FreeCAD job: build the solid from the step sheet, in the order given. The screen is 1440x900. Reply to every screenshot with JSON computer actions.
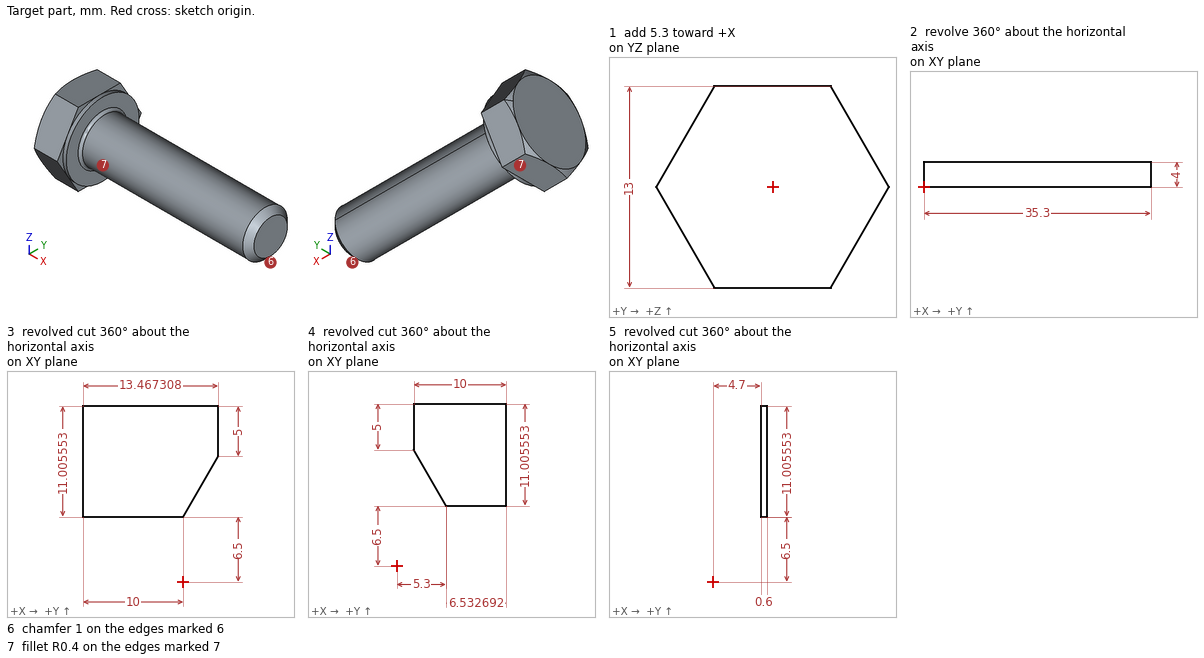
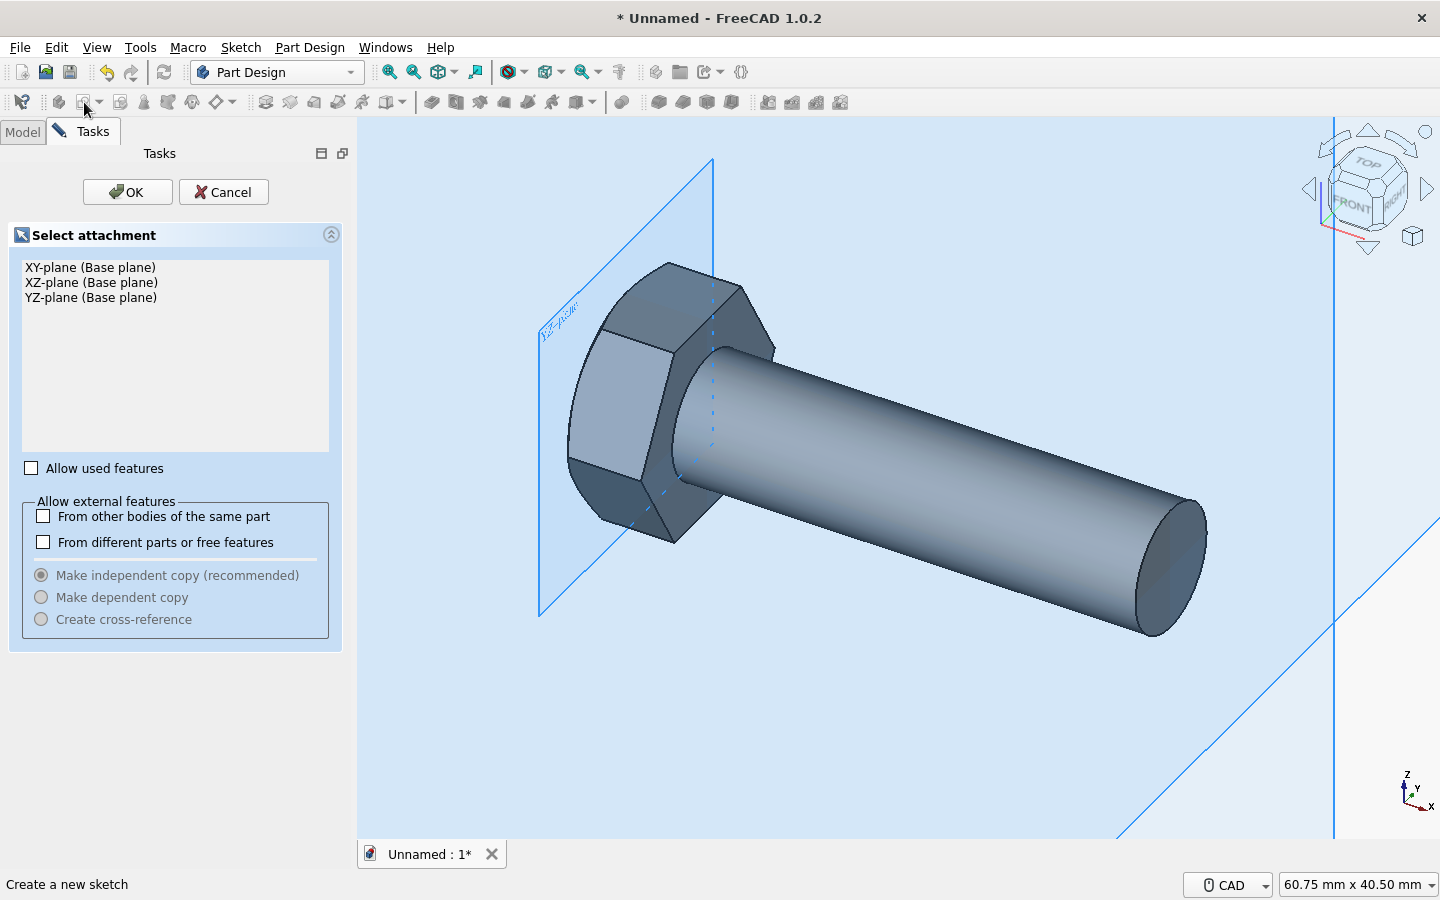
{"action": "left_click", "coordinate": [82, 268]}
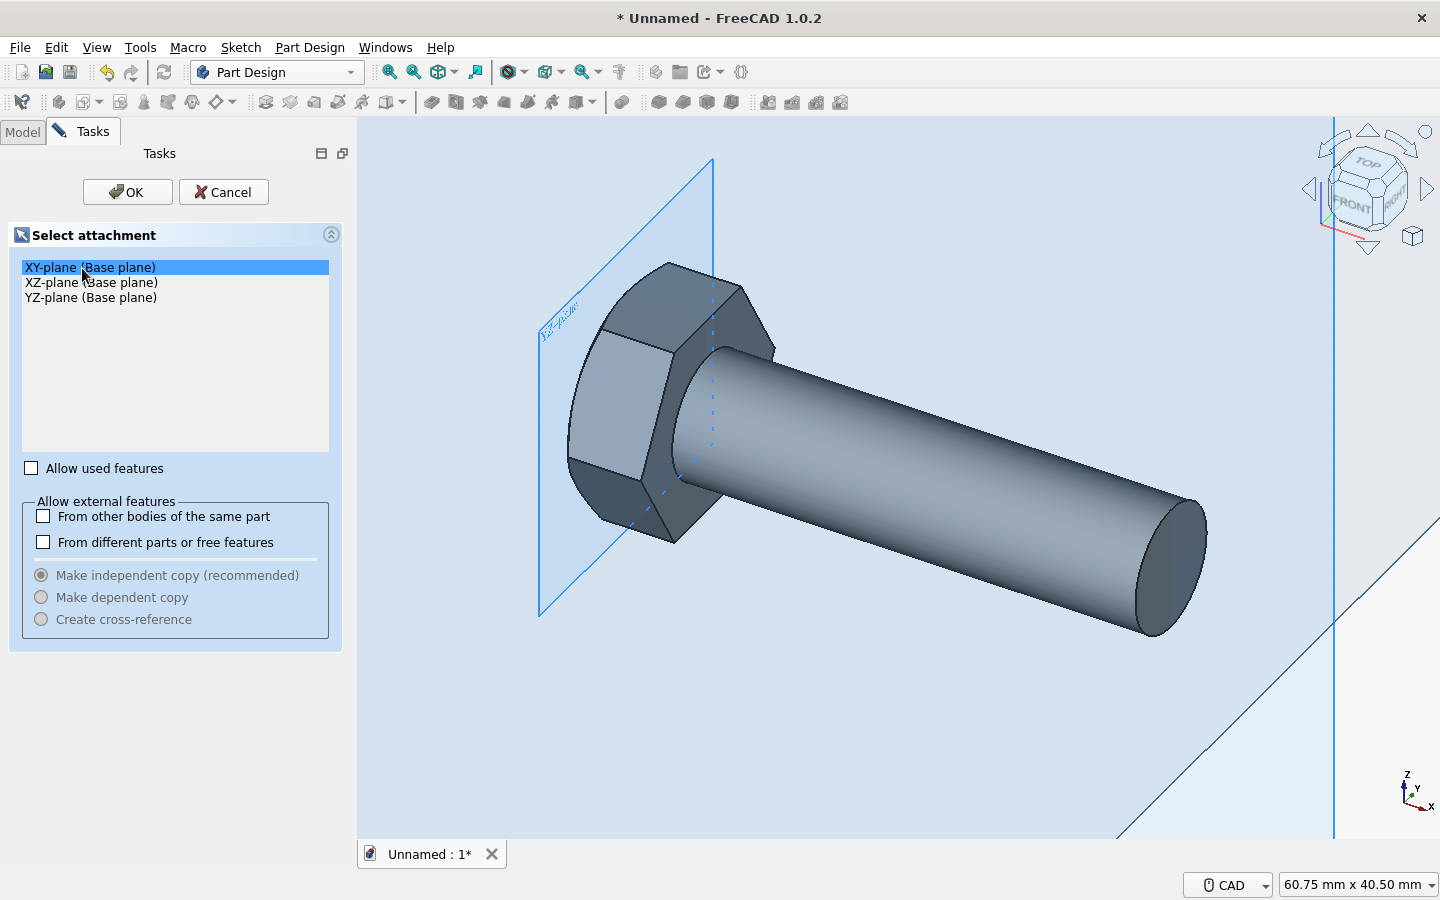
{"action": "left_click", "coordinate": [128, 192]}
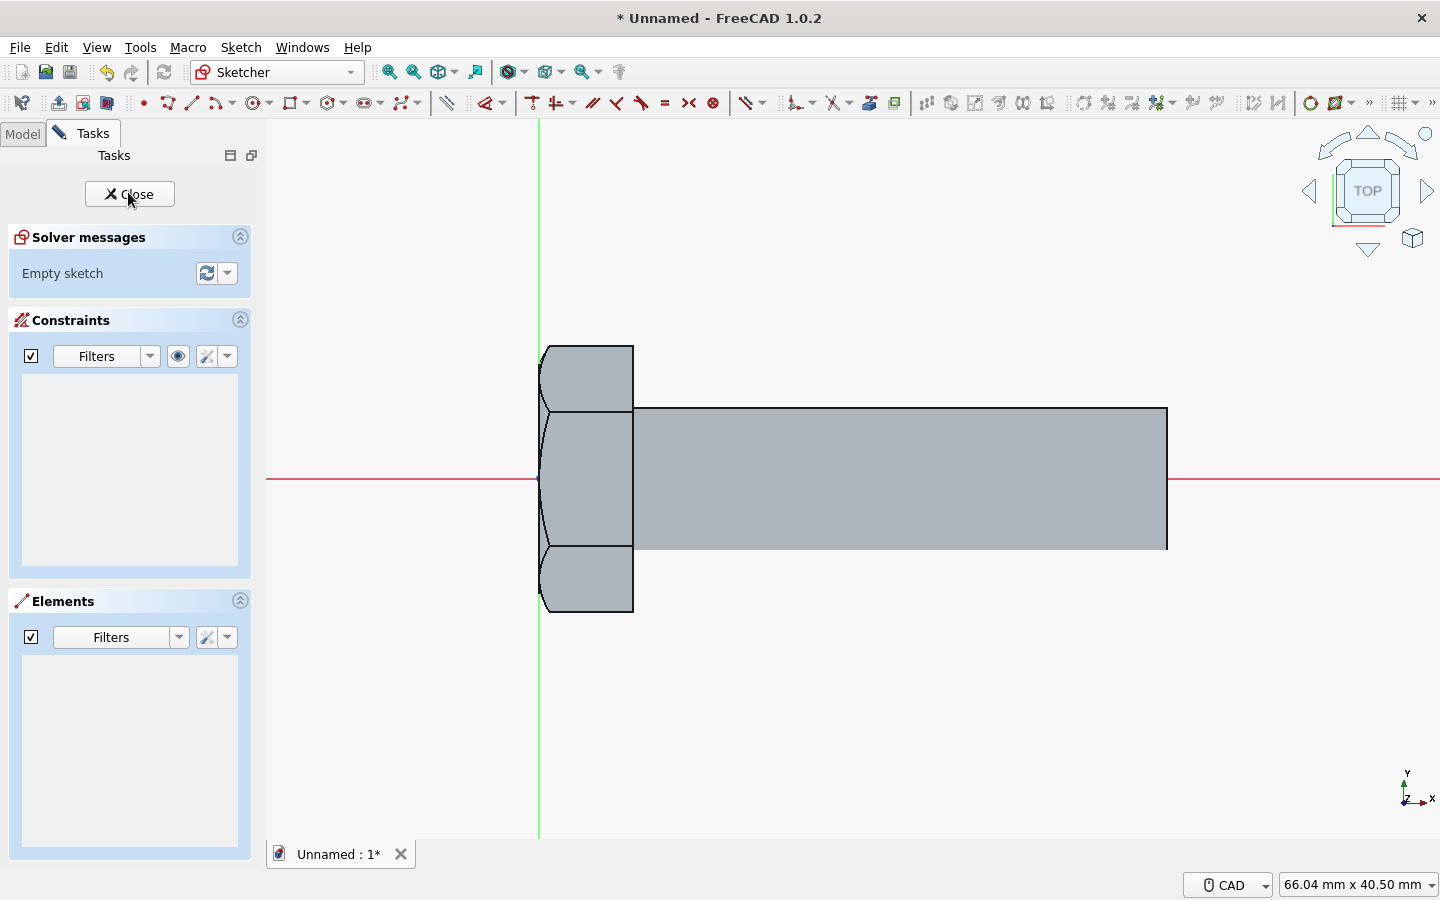
{"action": "left_click", "coordinate": [108, 104]}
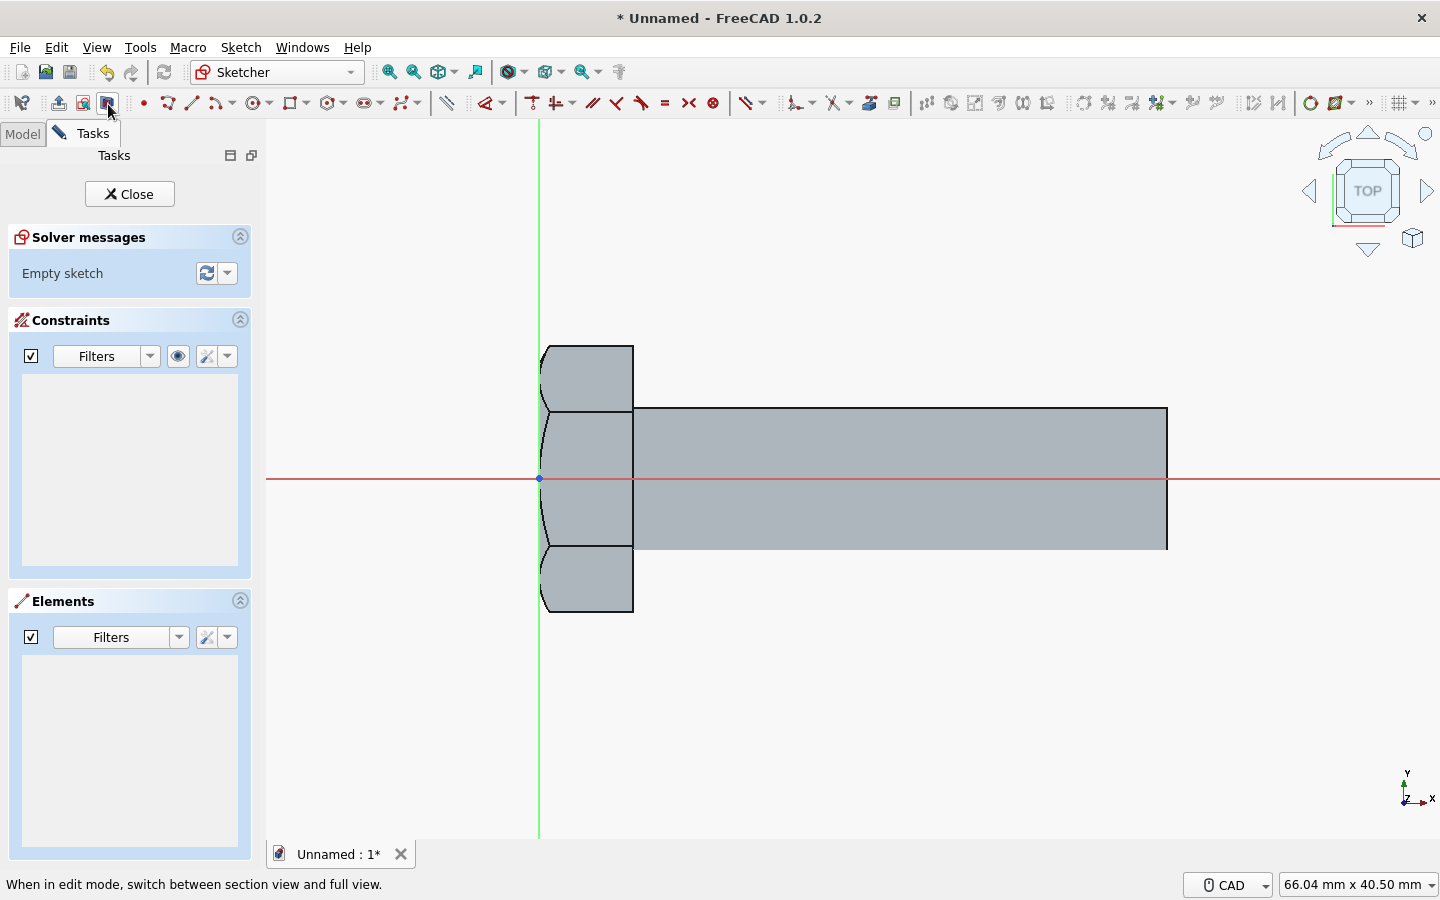
{"action": "scroll", "coordinate": [360, 147], "scroll_direction": "up", "scroll_amount": 2}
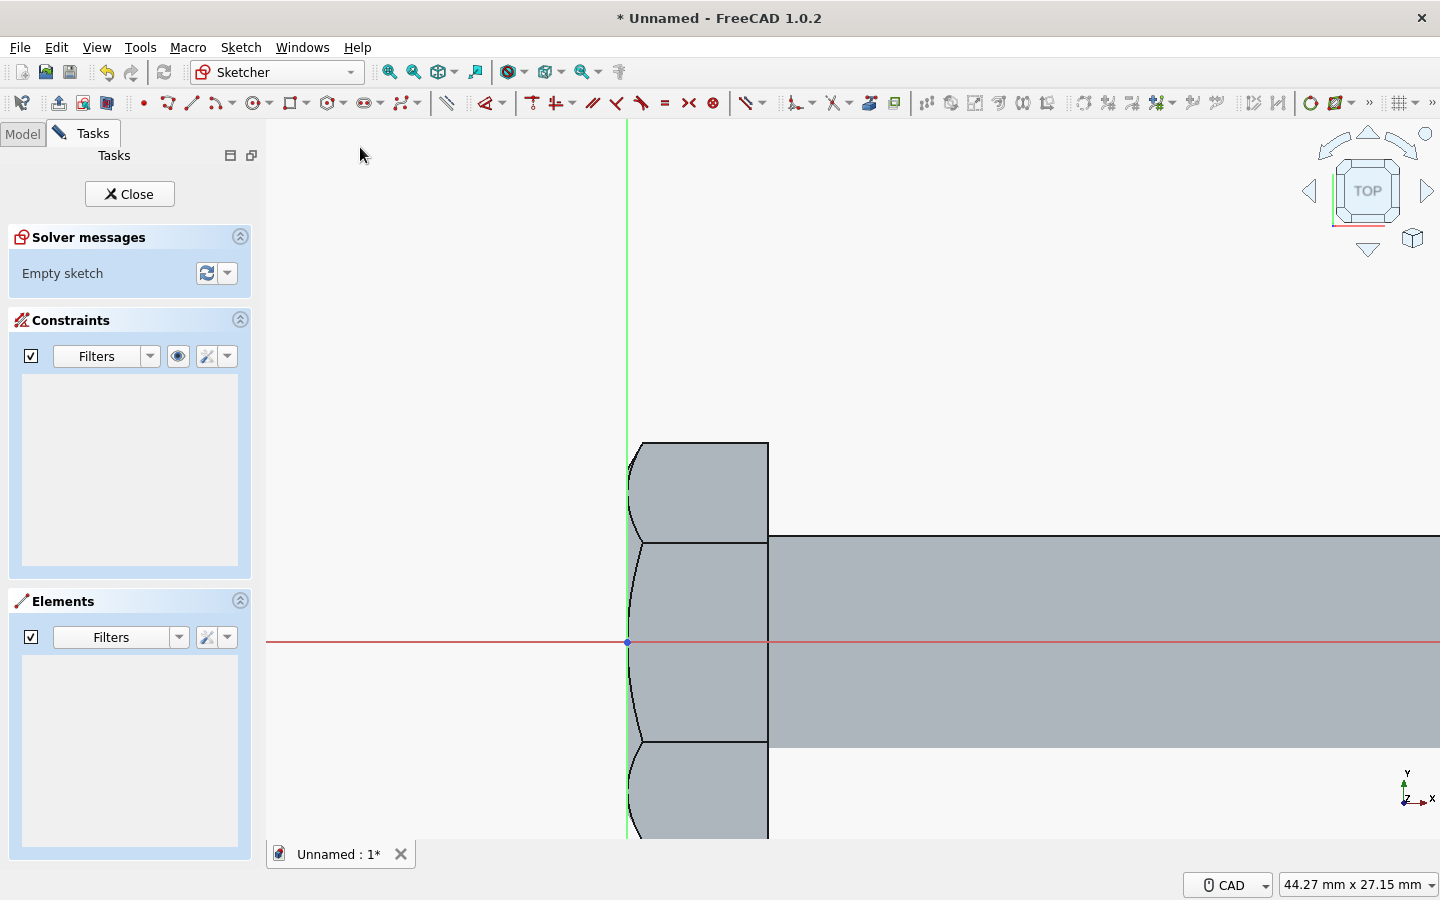
{"action": "key", "text": "g m"}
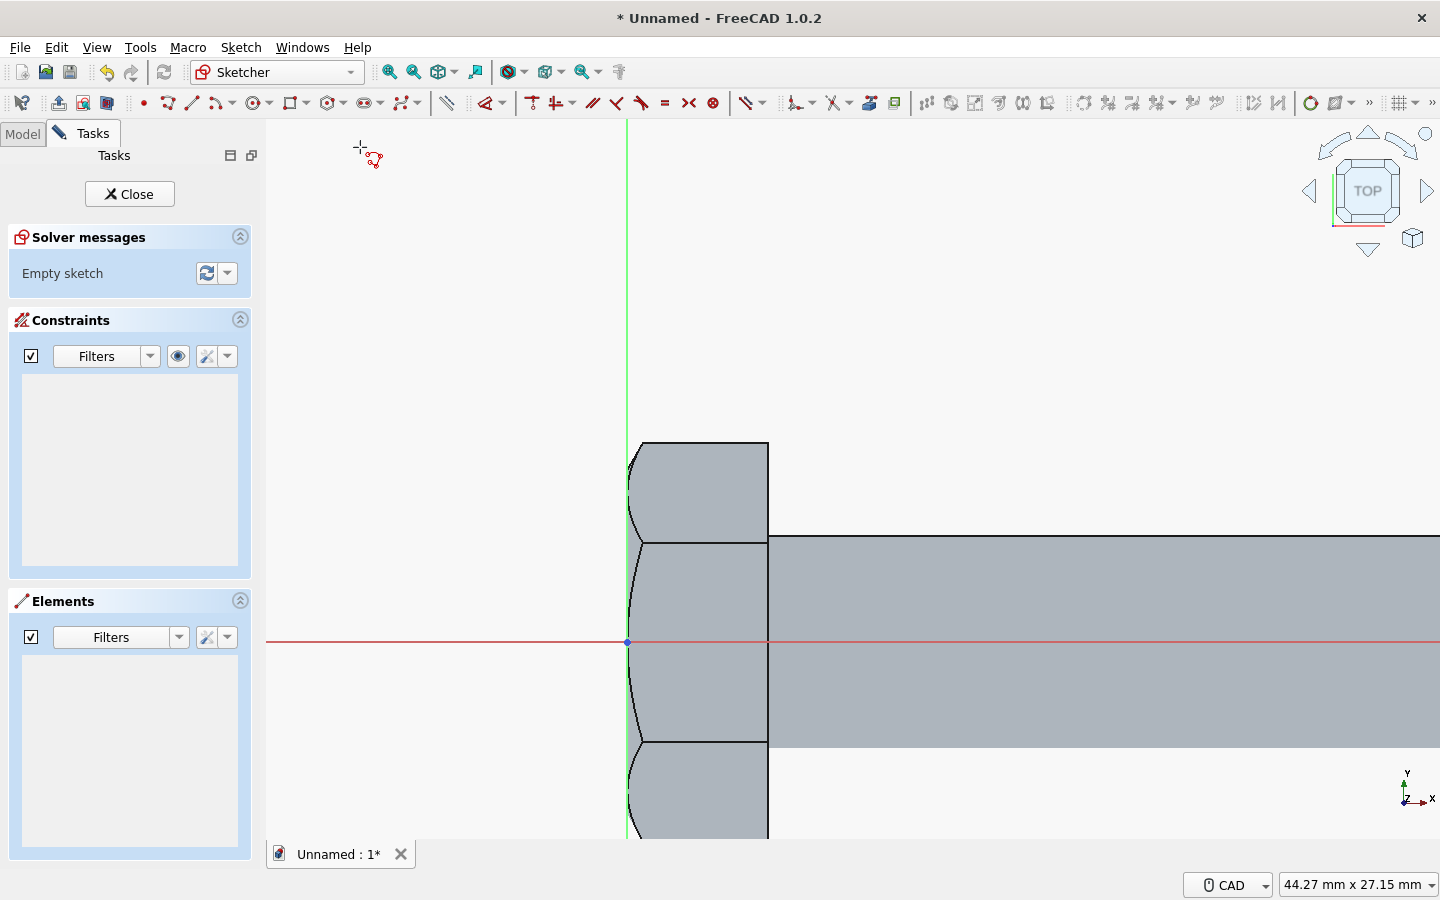
{"action": "left_click", "coordinate": [768, 470]}
{"action": "left_click", "coordinate": [941, 470]}
{"action": "left_click", "coordinate": [941, 178]}
{"action": "left_click", "coordinate": [676, 178]}
{"action": "left_click", "coordinate": [676, 311]}
{"action": "left_click", "coordinate": [768, 471]}
{"action": "key", "text": "Escape"}
{"action": "key", "text": "Escape"}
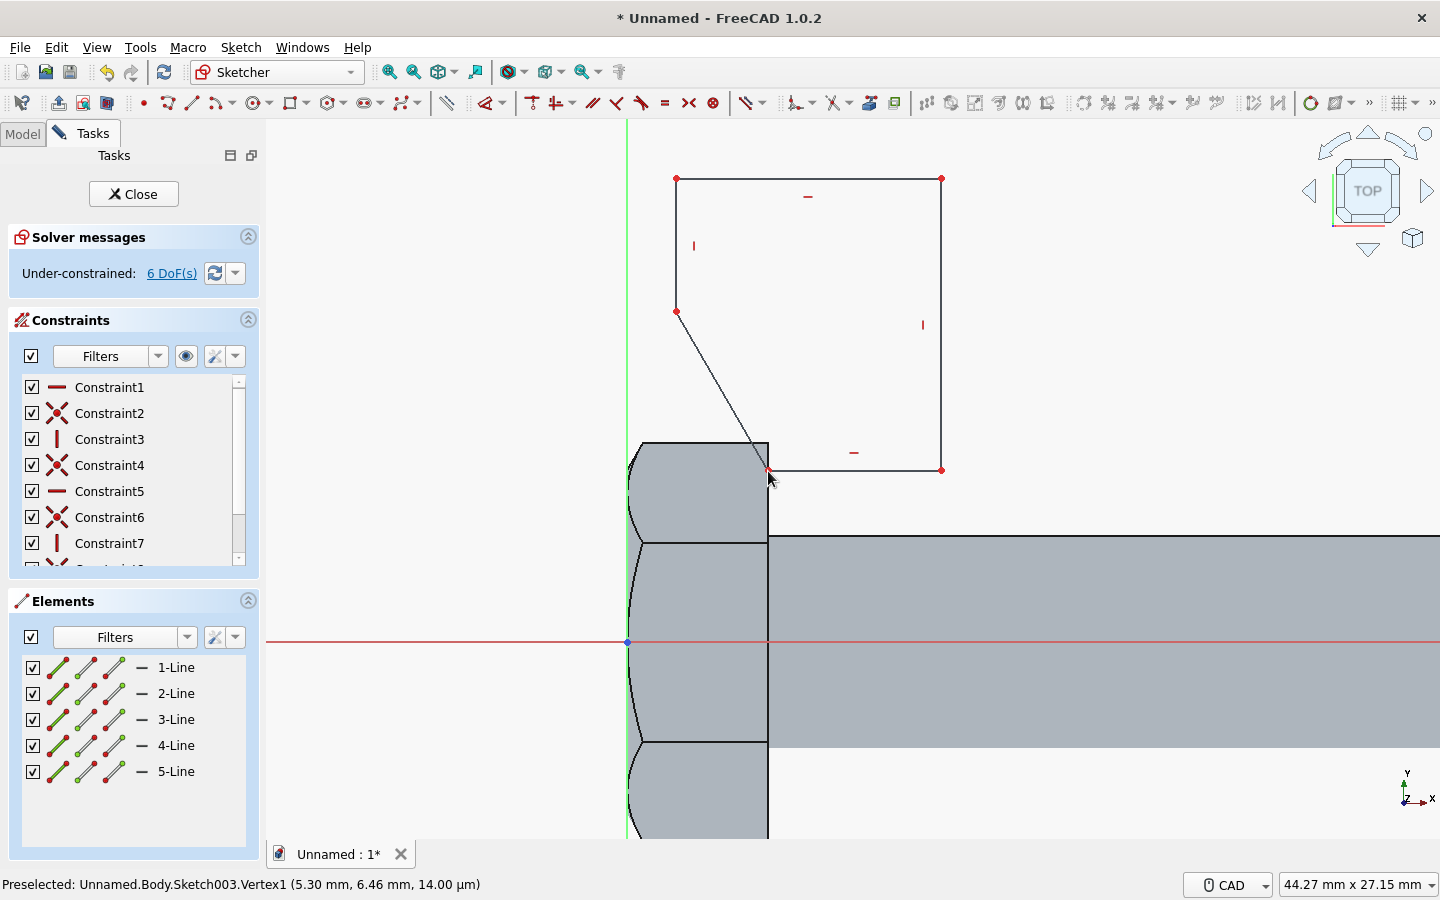
{"action": "key", "text": "d"}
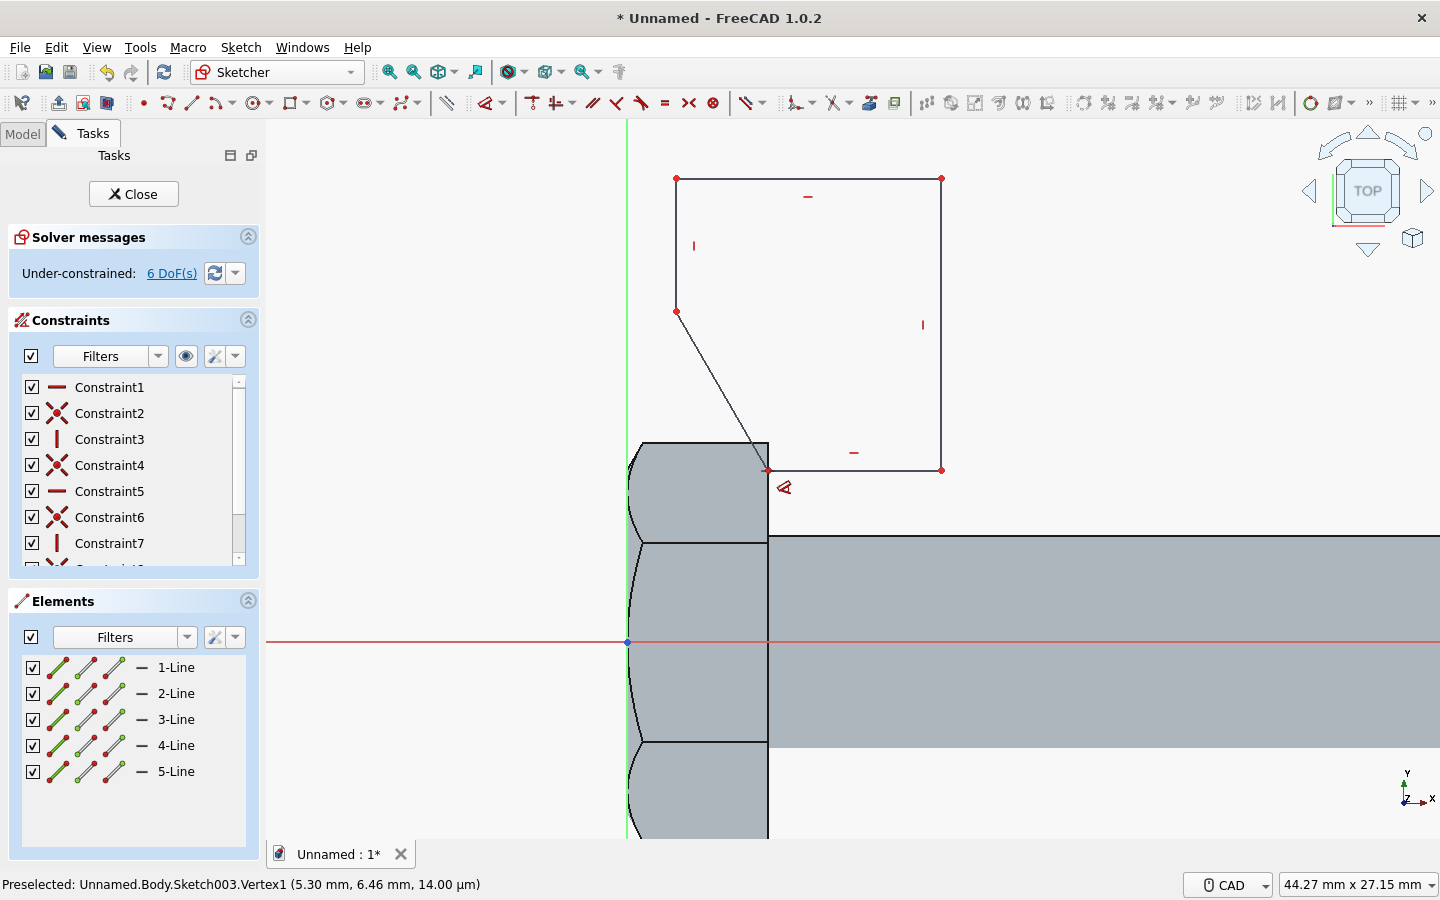
{"action": "left_click", "coordinate": [676, 219]}
{"action": "left_click", "coordinate": [642, 245]}